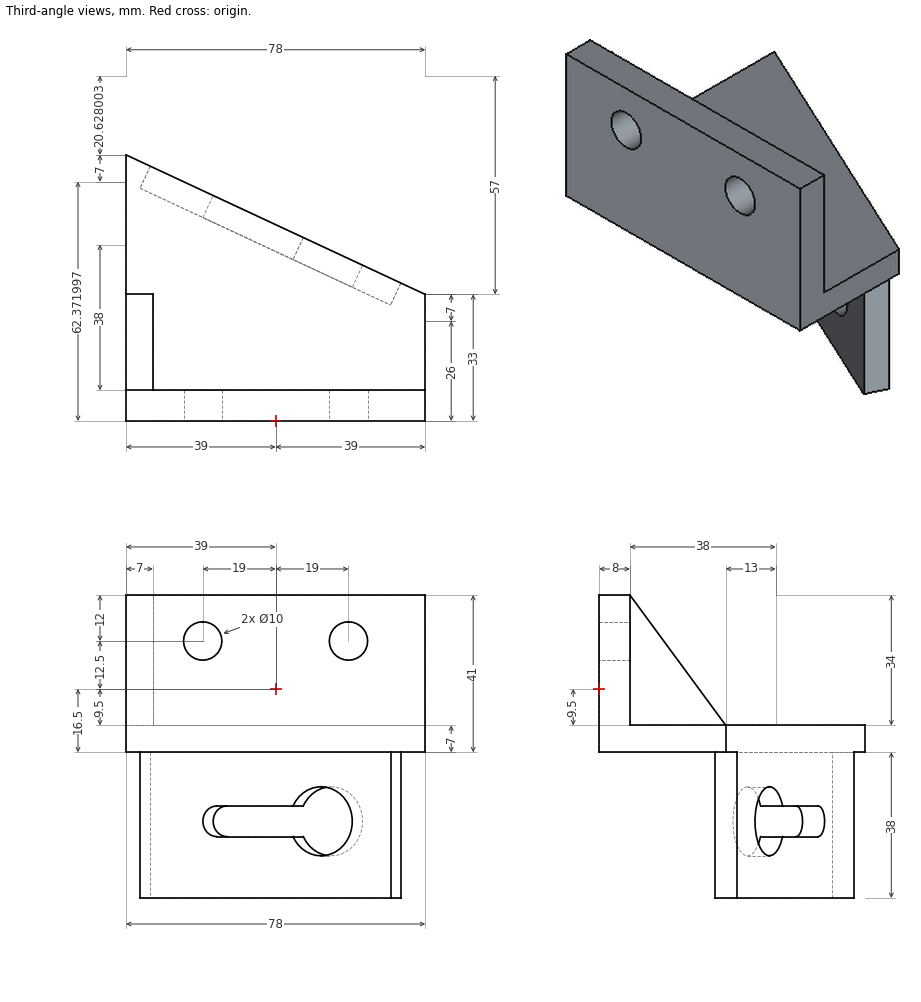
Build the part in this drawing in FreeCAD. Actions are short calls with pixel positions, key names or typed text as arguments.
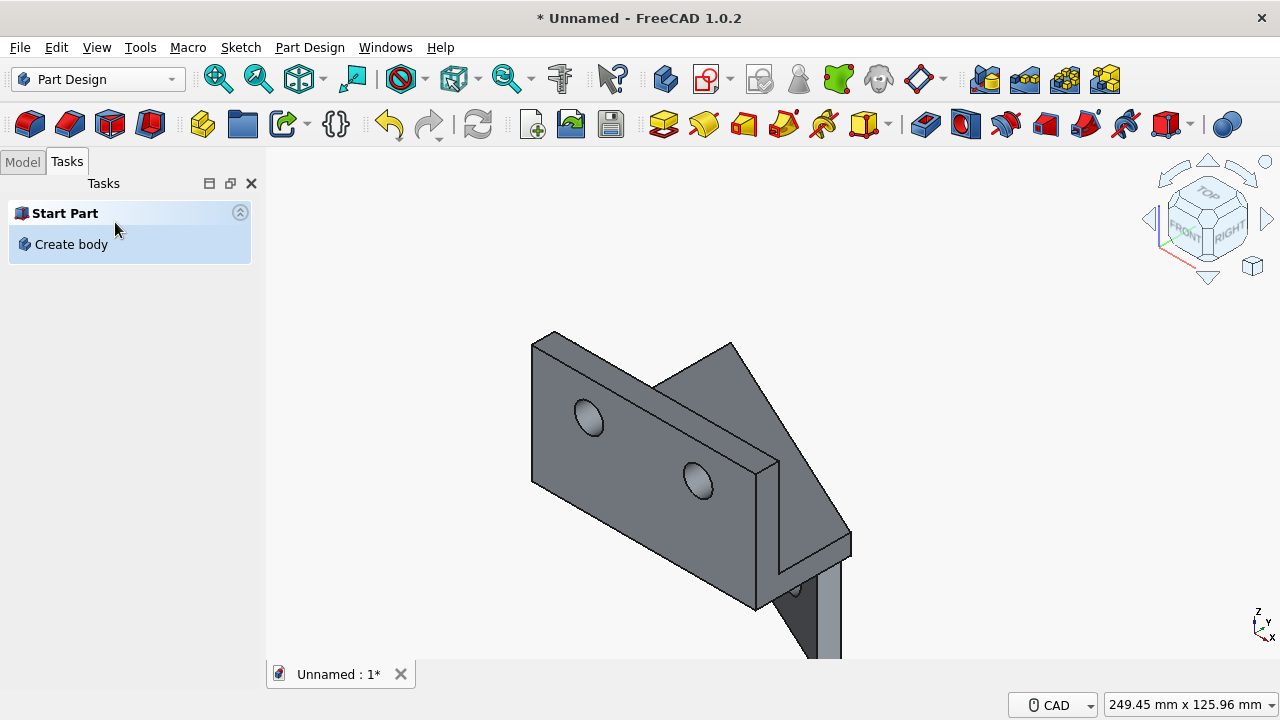
click(220, 80)